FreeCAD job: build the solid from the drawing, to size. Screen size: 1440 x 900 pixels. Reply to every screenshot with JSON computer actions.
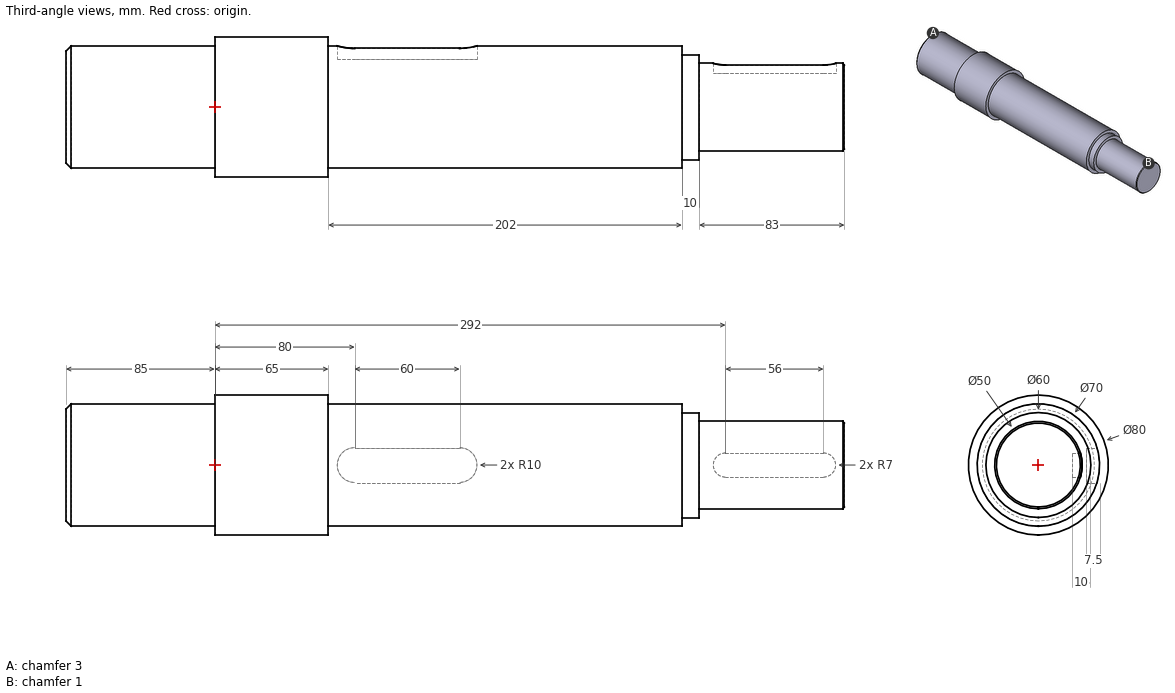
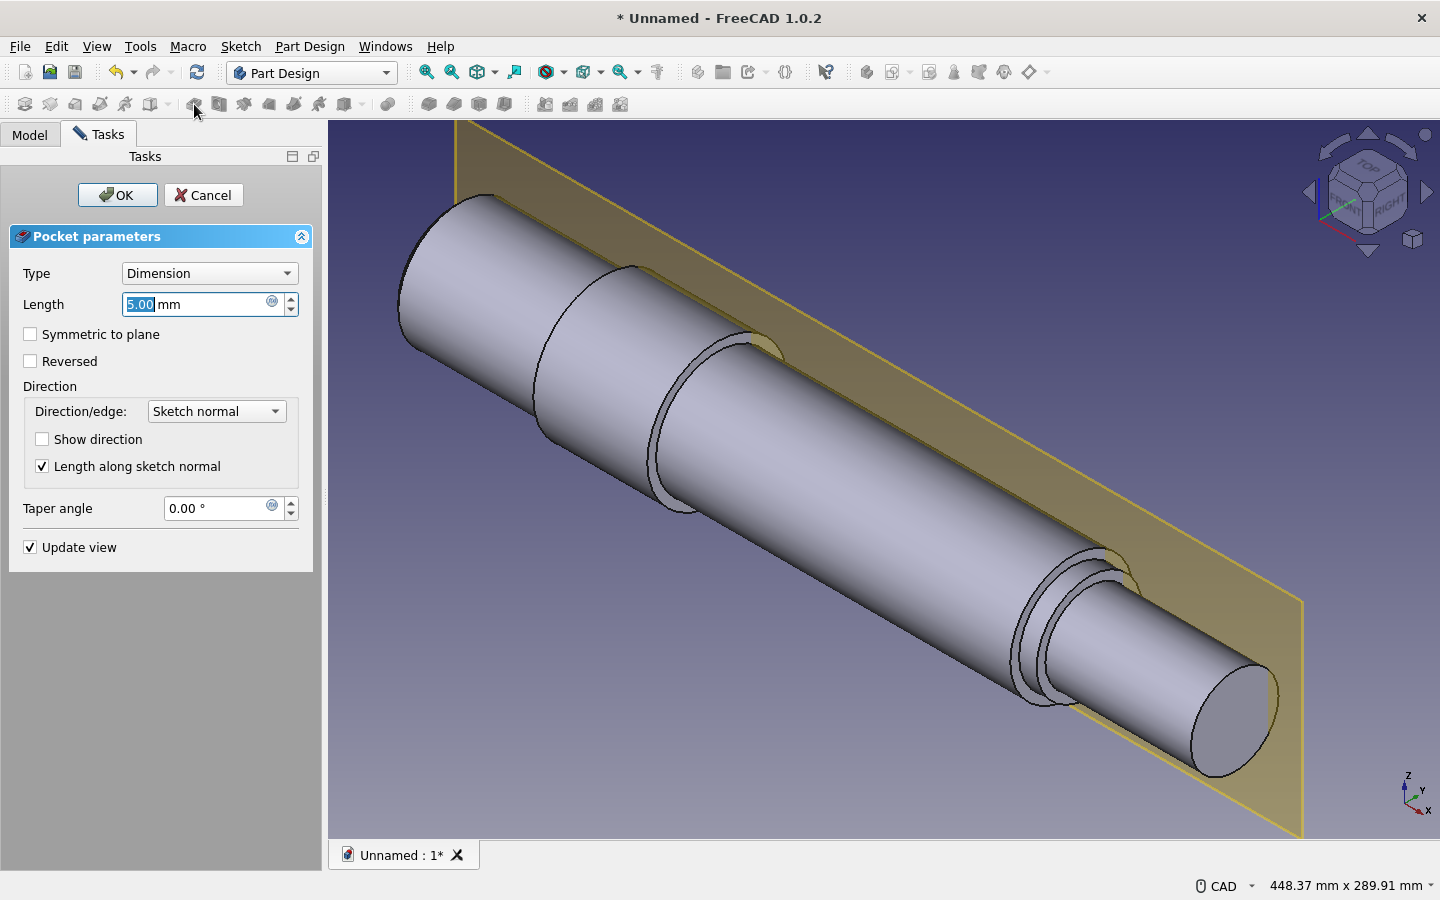
{"action": "type", "text": "10"}
{"action": "key", "text": "Tab"}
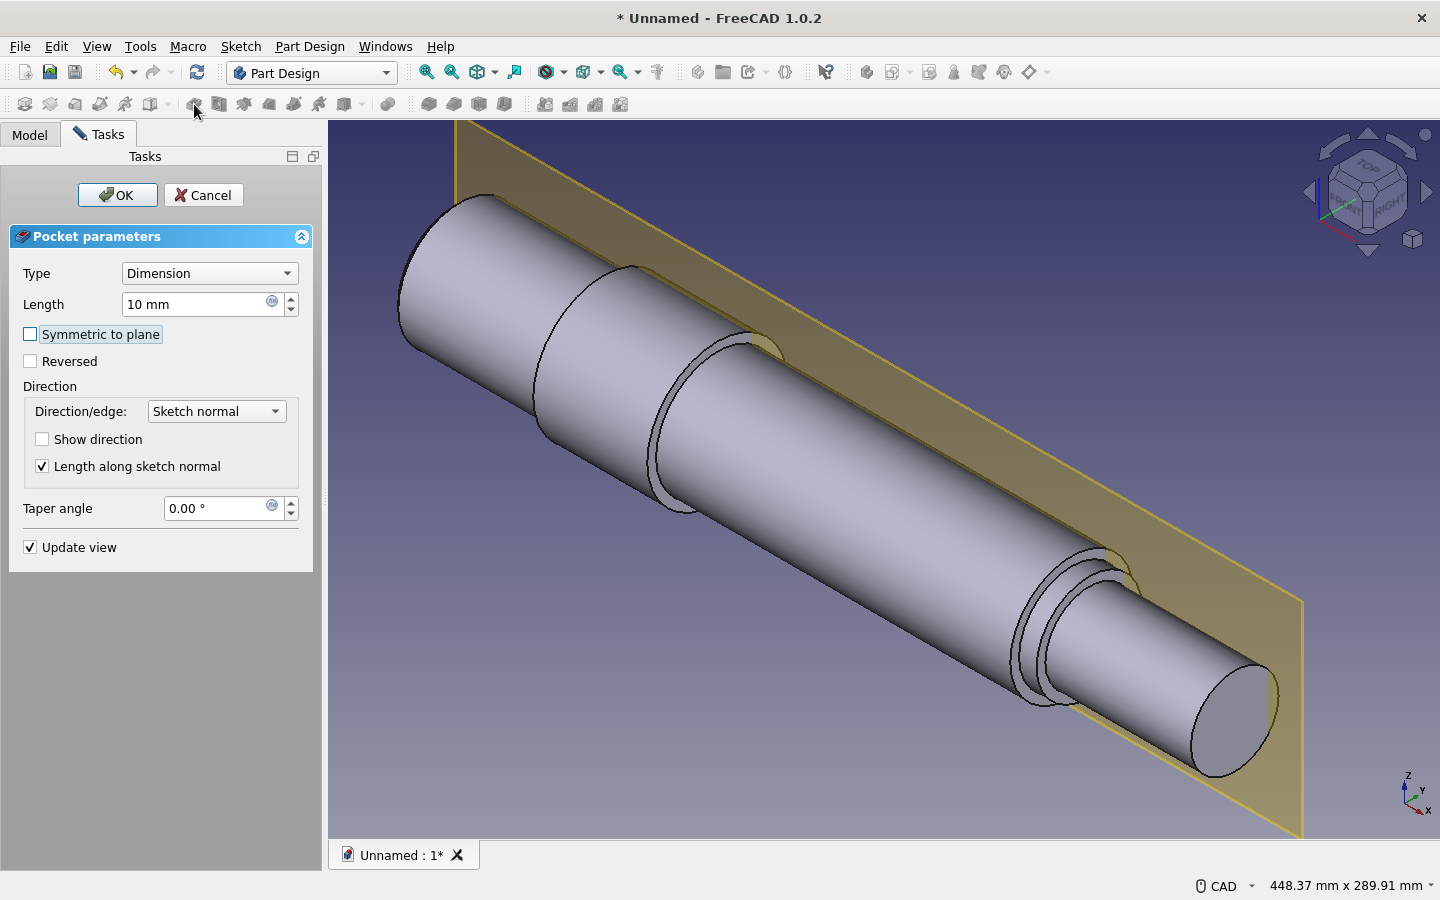
{"action": "left_click", "coordinate": [118, 195]}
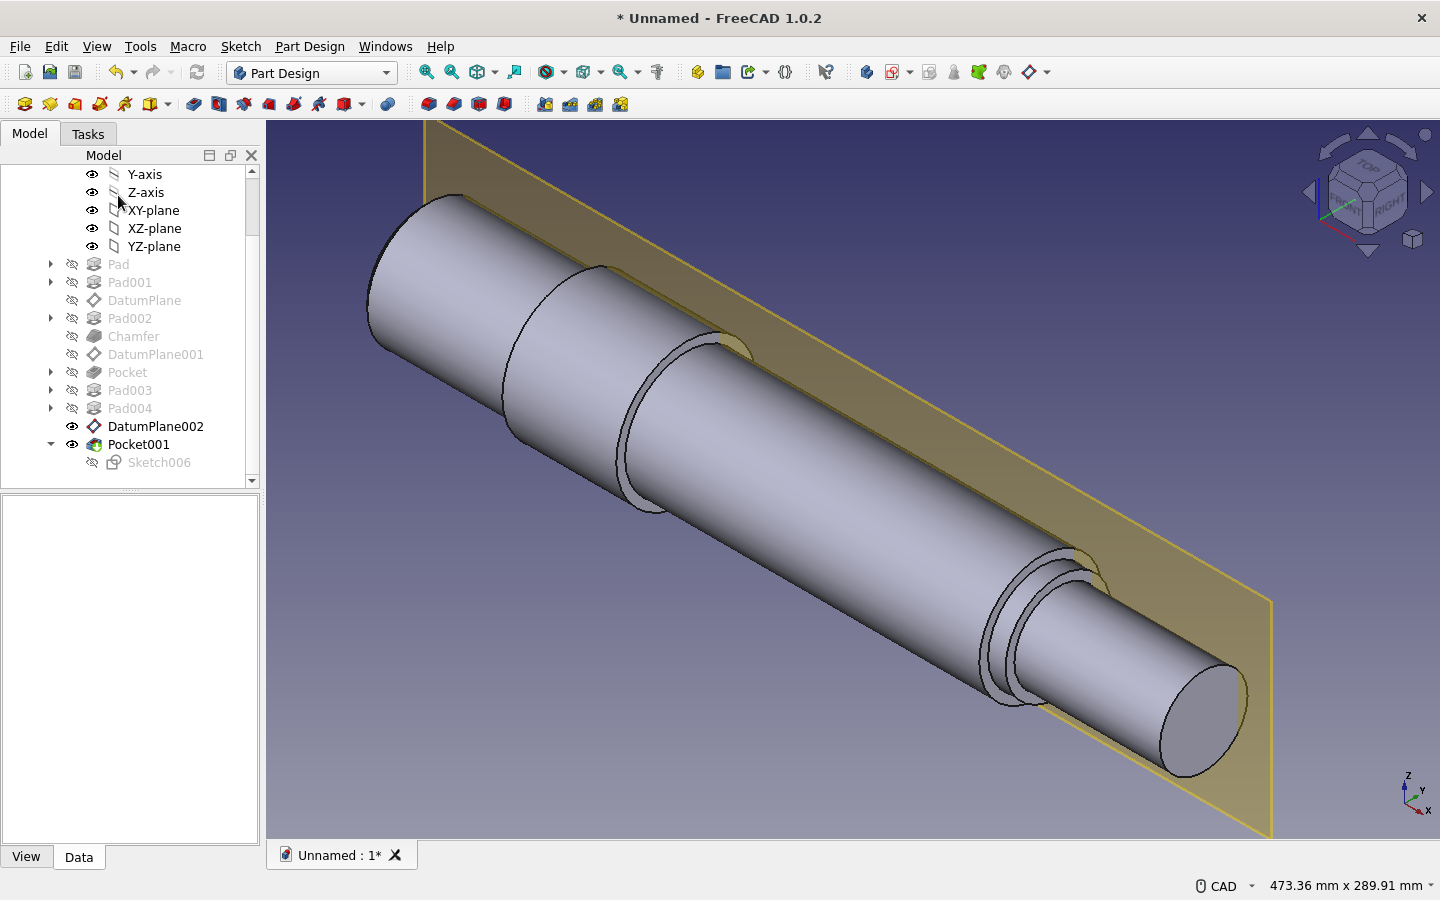
{"action": "left_click", "coordinate": [117, 426]}
{"action": "key", "text": "space"}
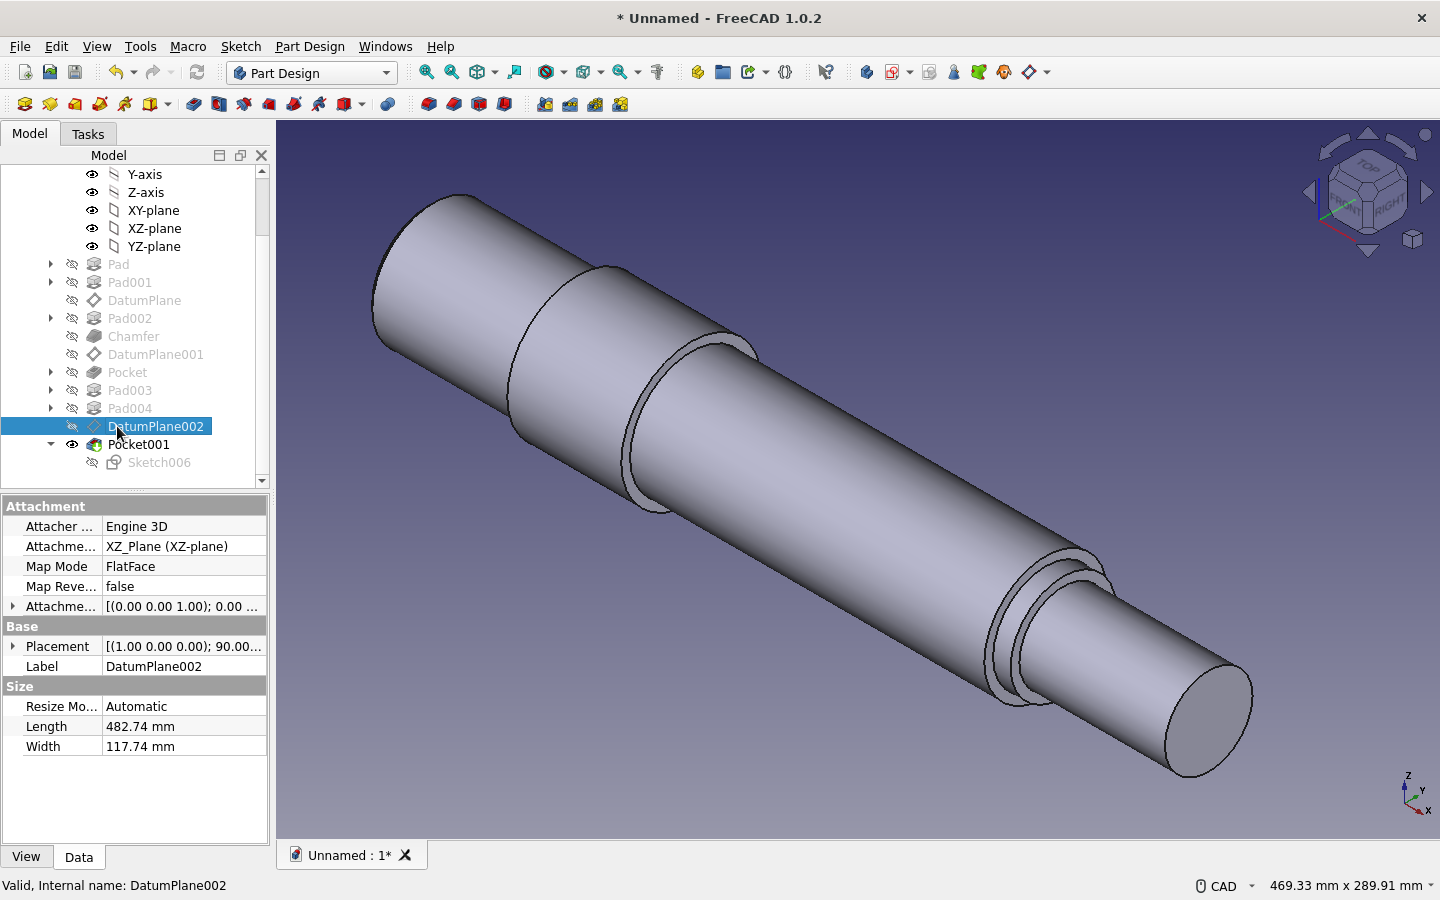
{"action": "key", "text": "v f"}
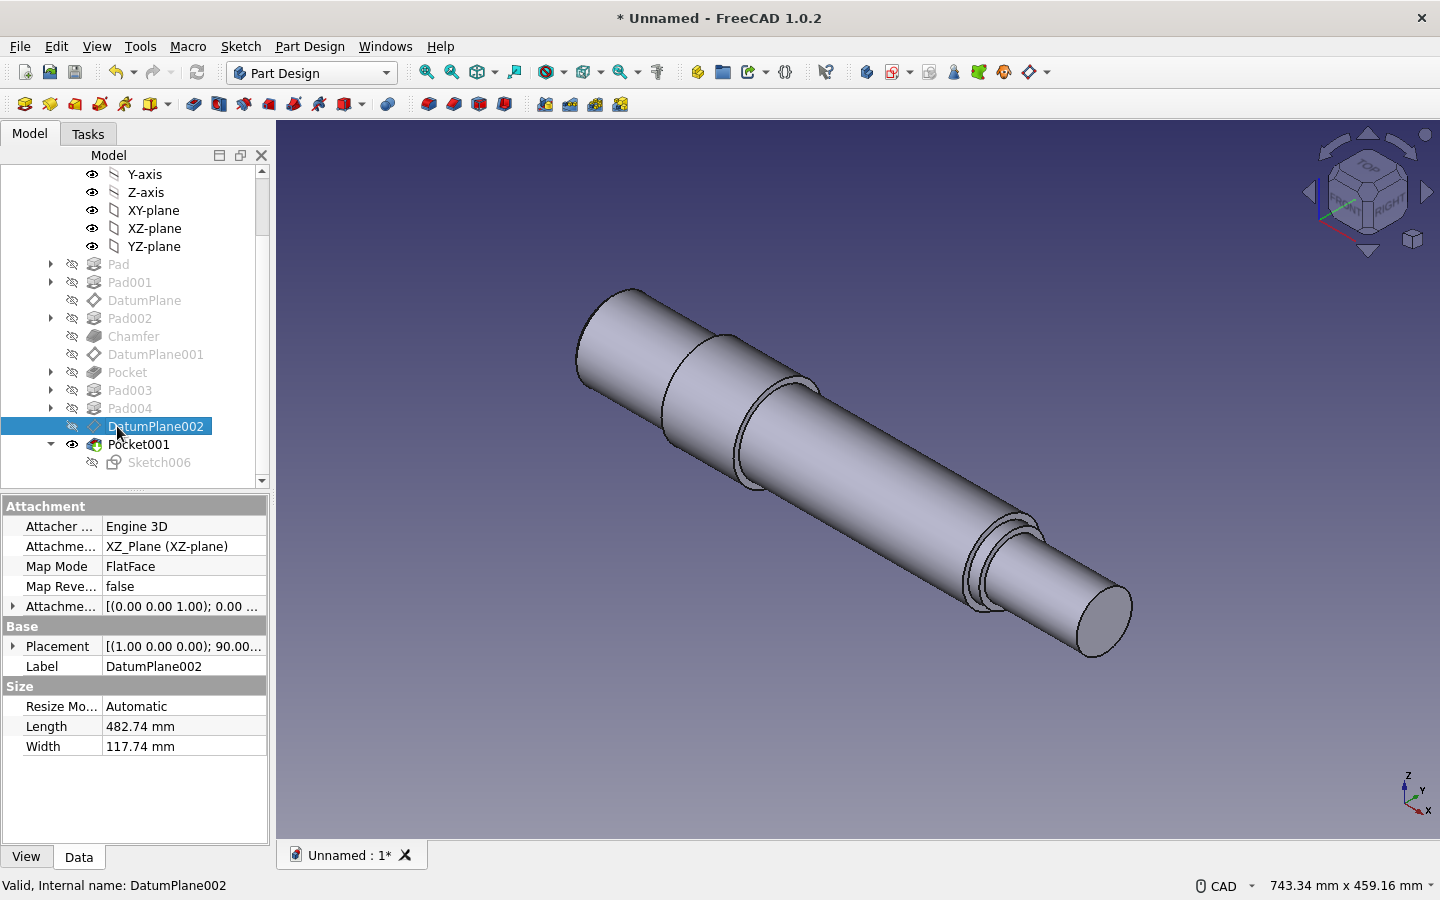
{"action": "left_click", "coordinate": [1077, 637]}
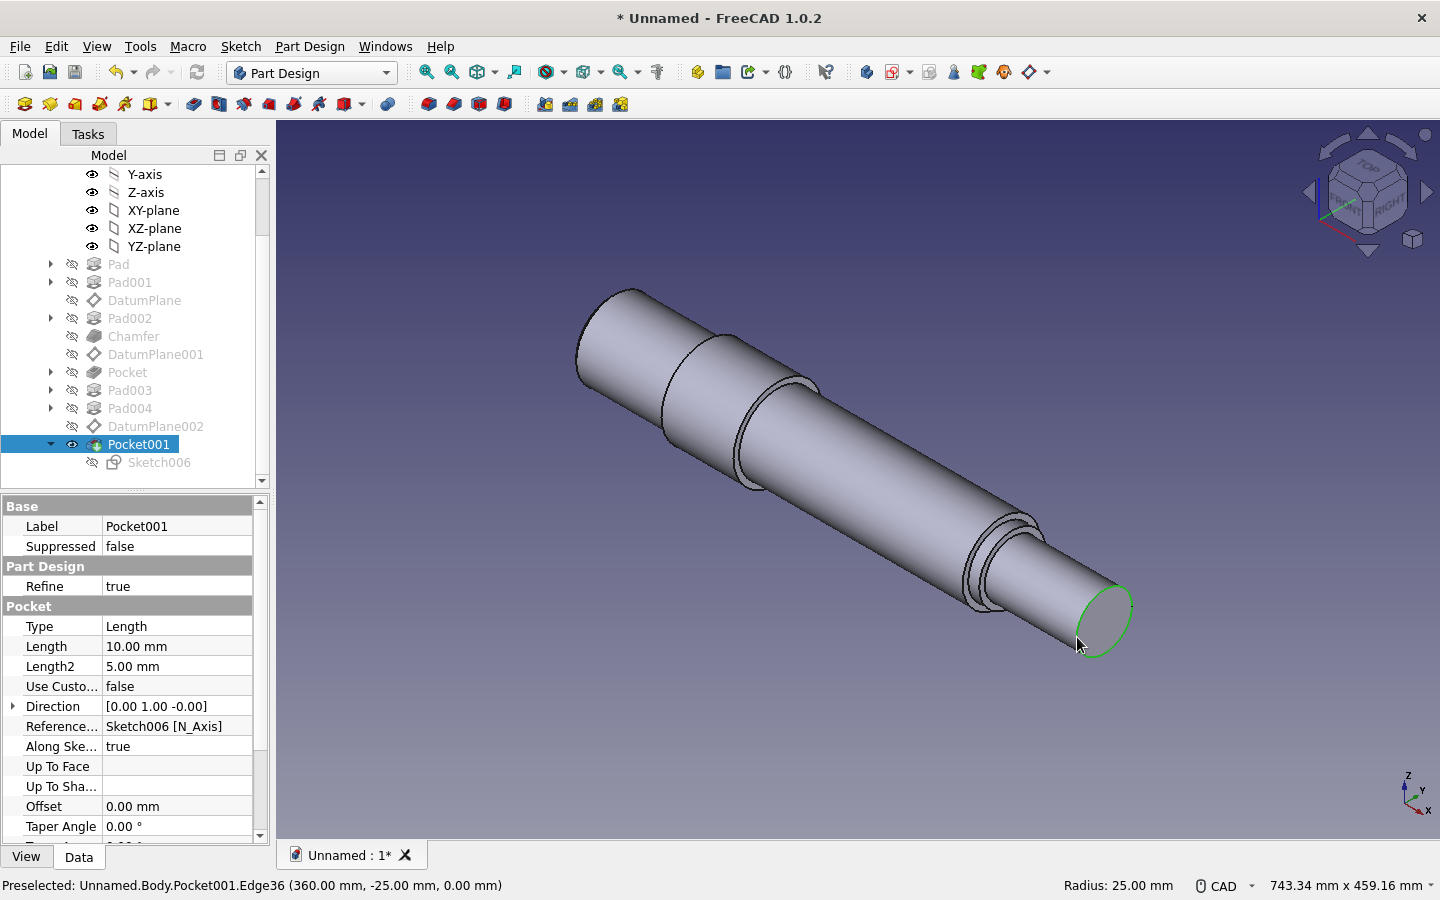
{"action": "left_click", "coordinate": [454, 104]}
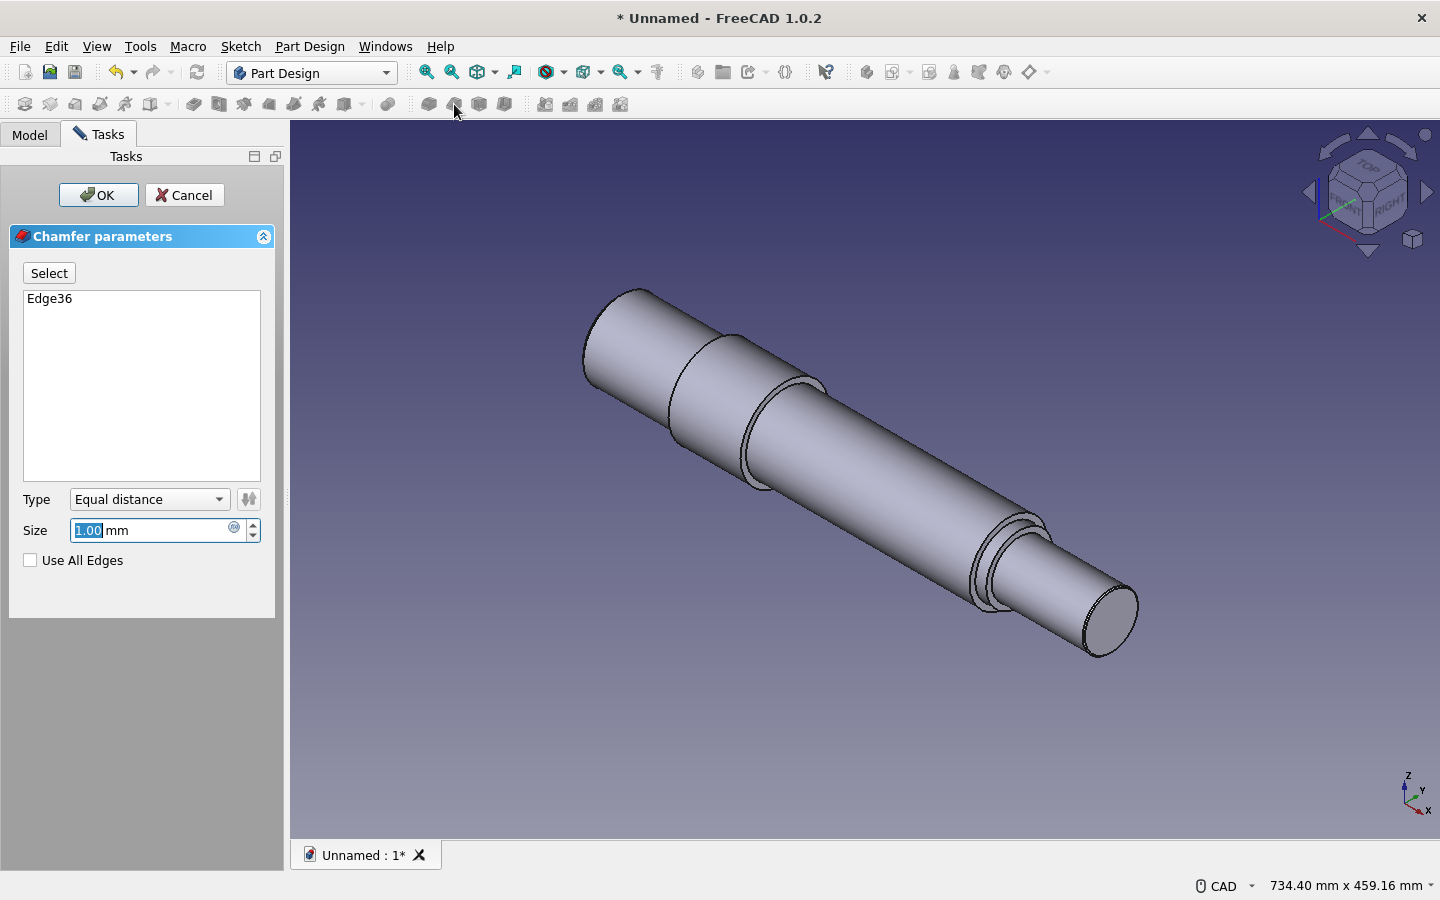
{"action": "type", "text": "1"}
{"action": "key", "text": "Tab"}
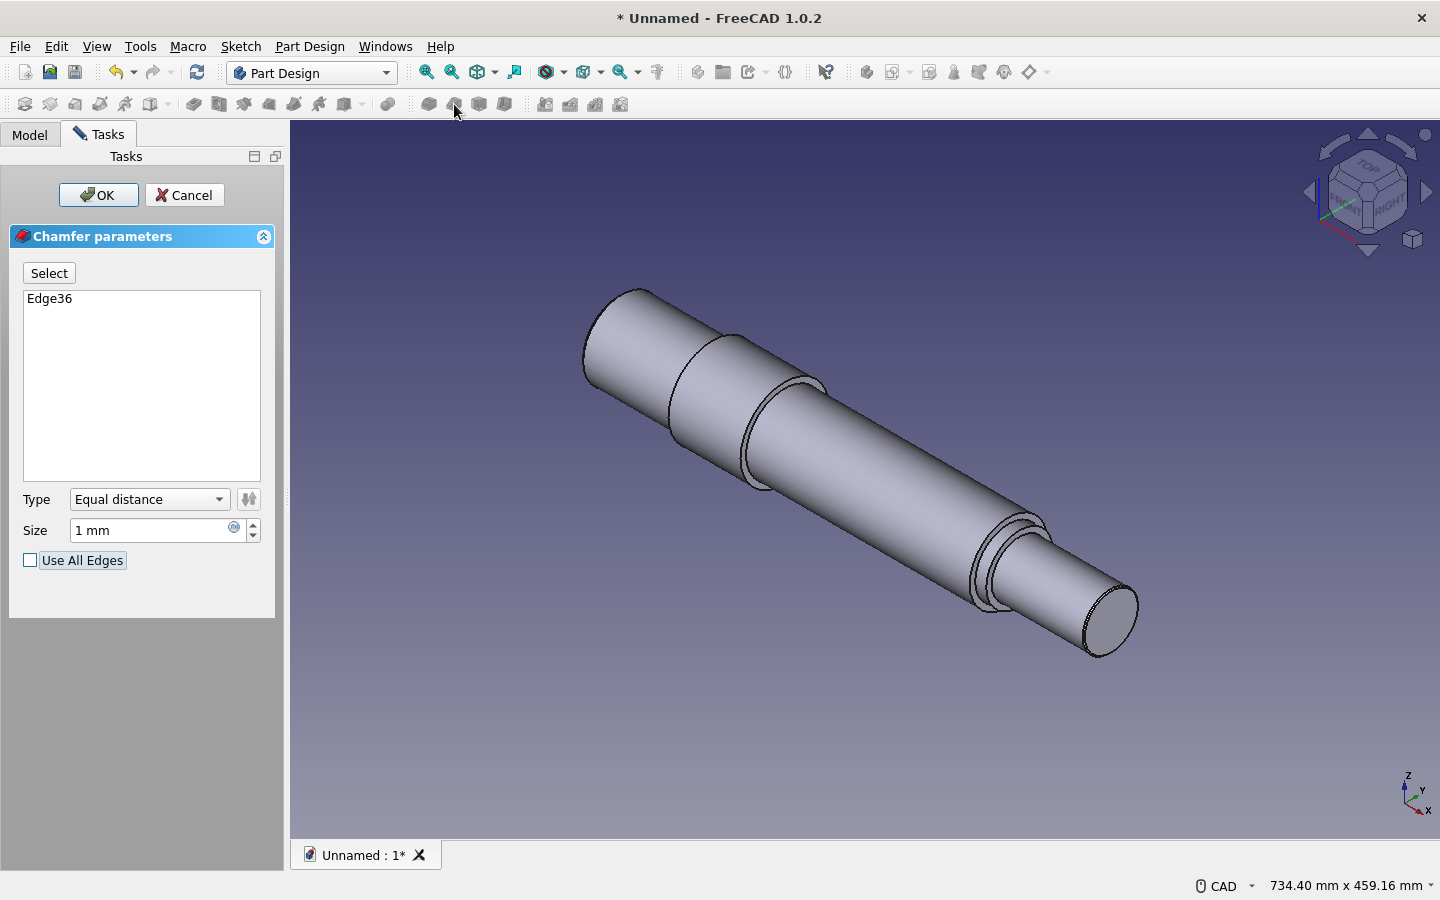
{"action": "left_click", "coordinate": [99, 195]}